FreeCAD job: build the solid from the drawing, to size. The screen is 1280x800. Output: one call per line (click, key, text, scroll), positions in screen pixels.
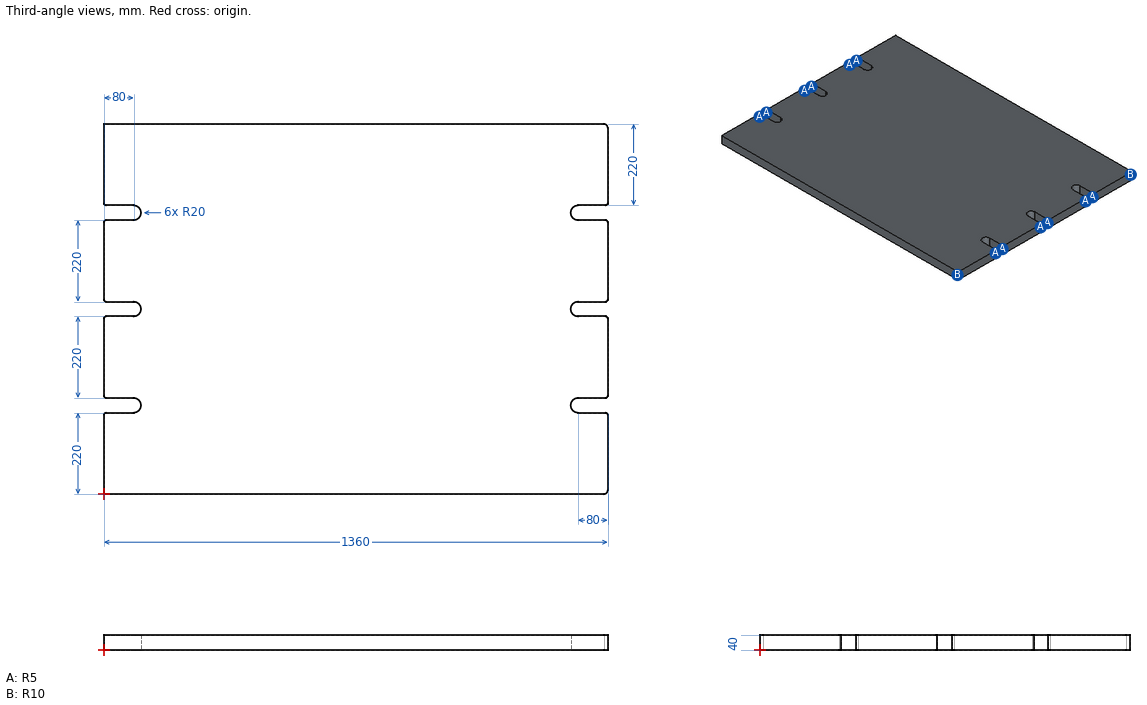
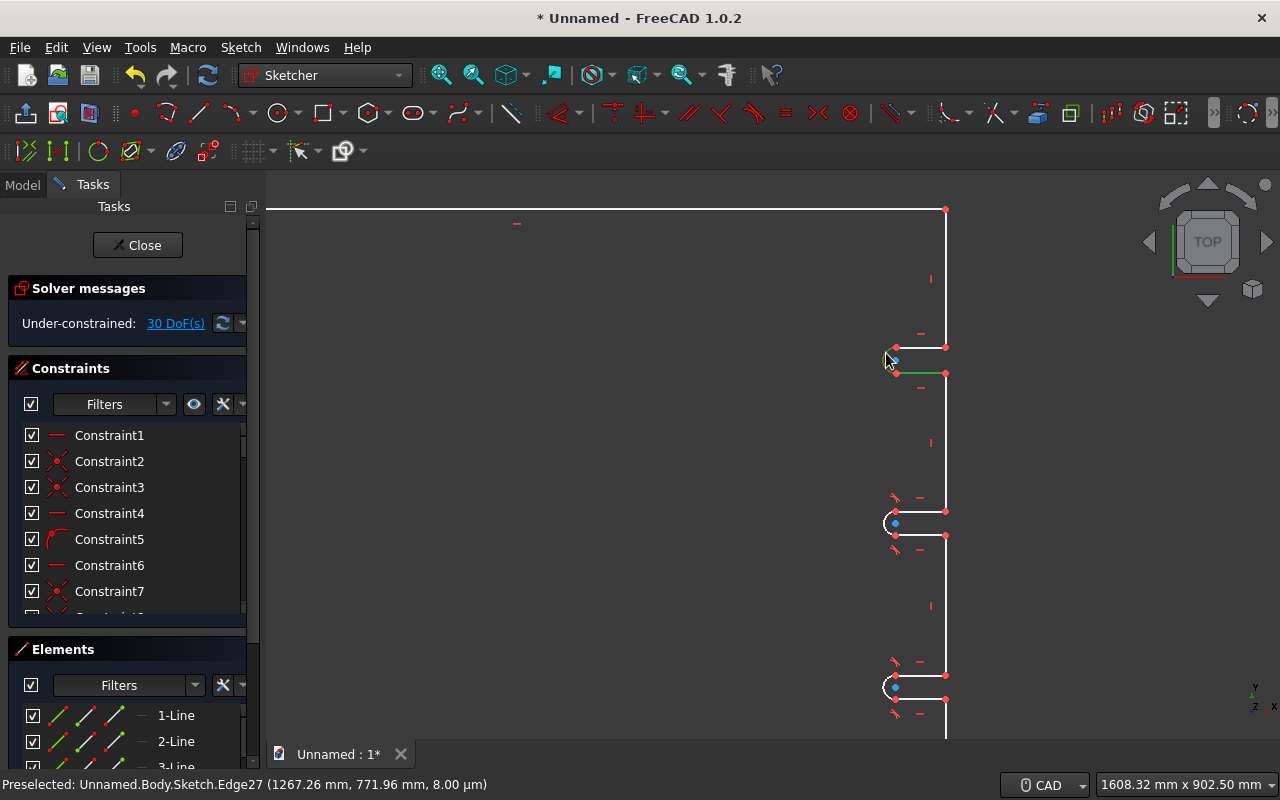
click(754, 114)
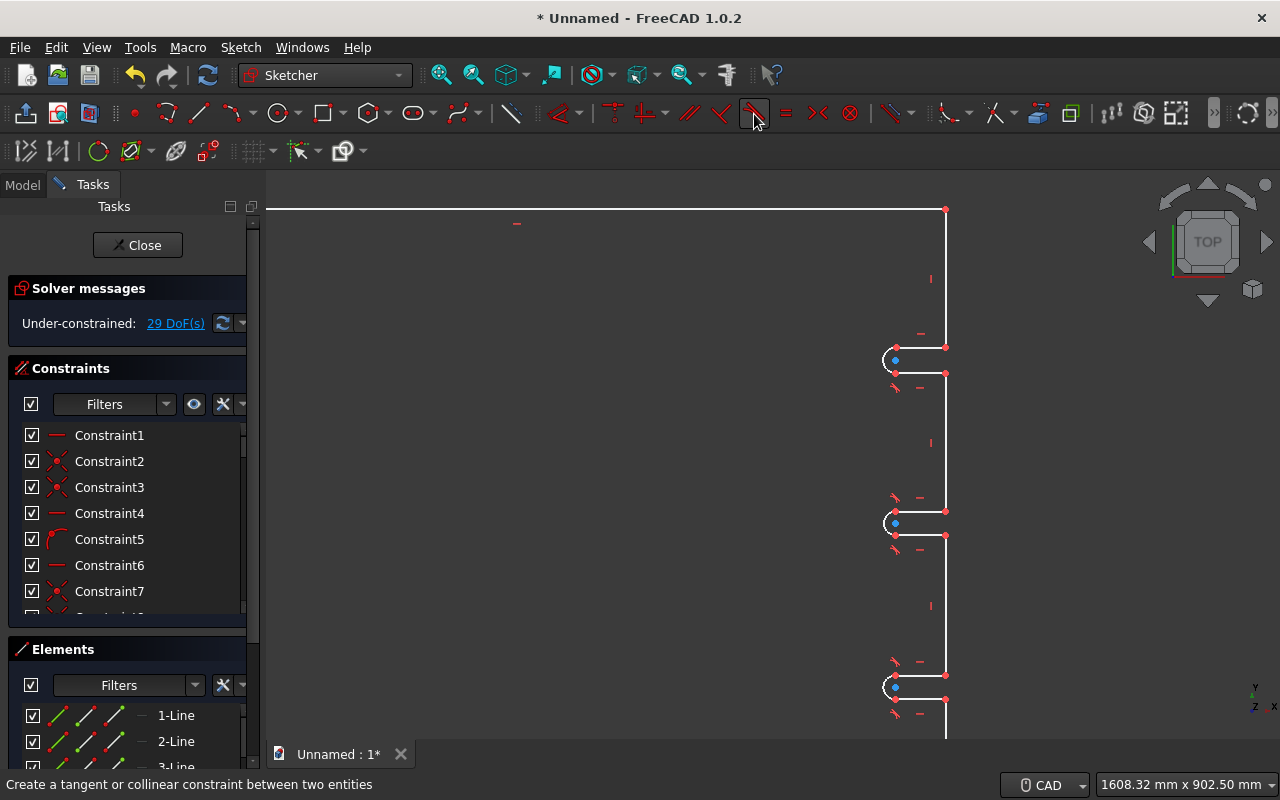
click(911, 348)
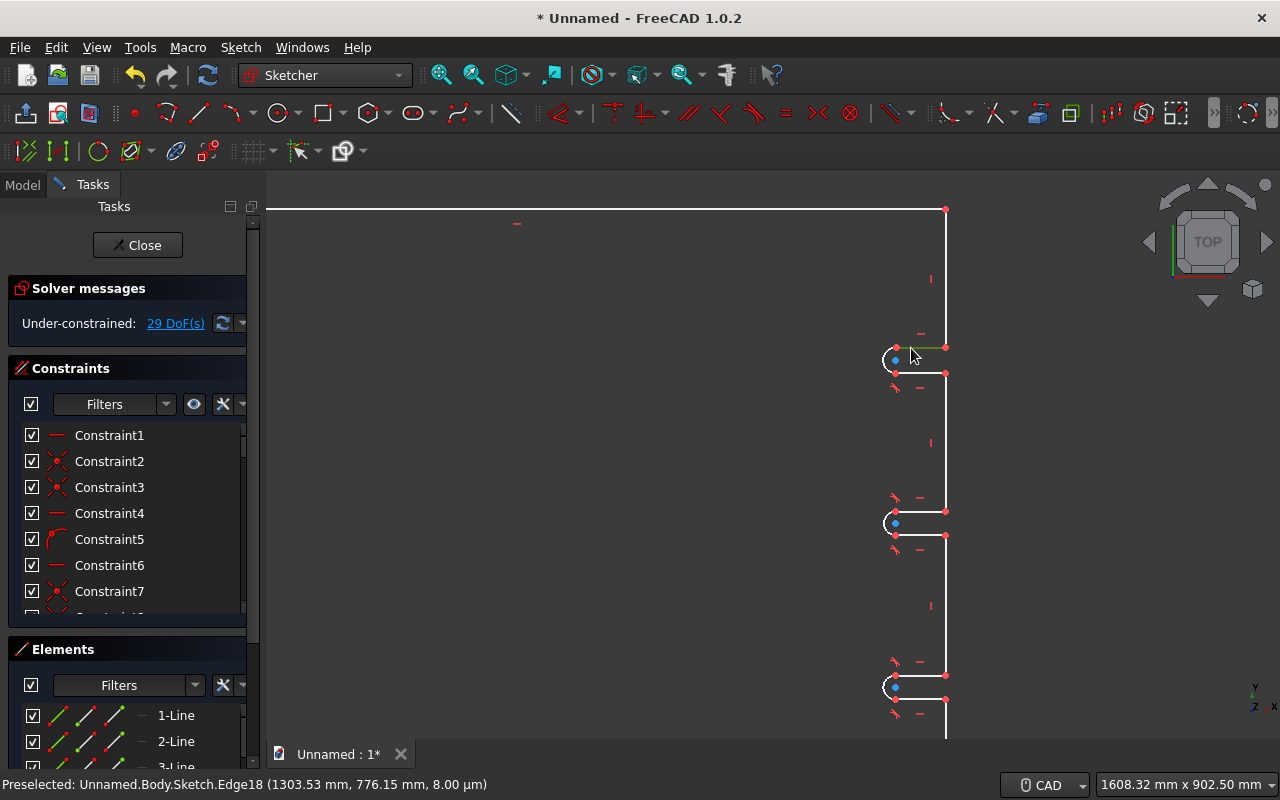
click(886, 352)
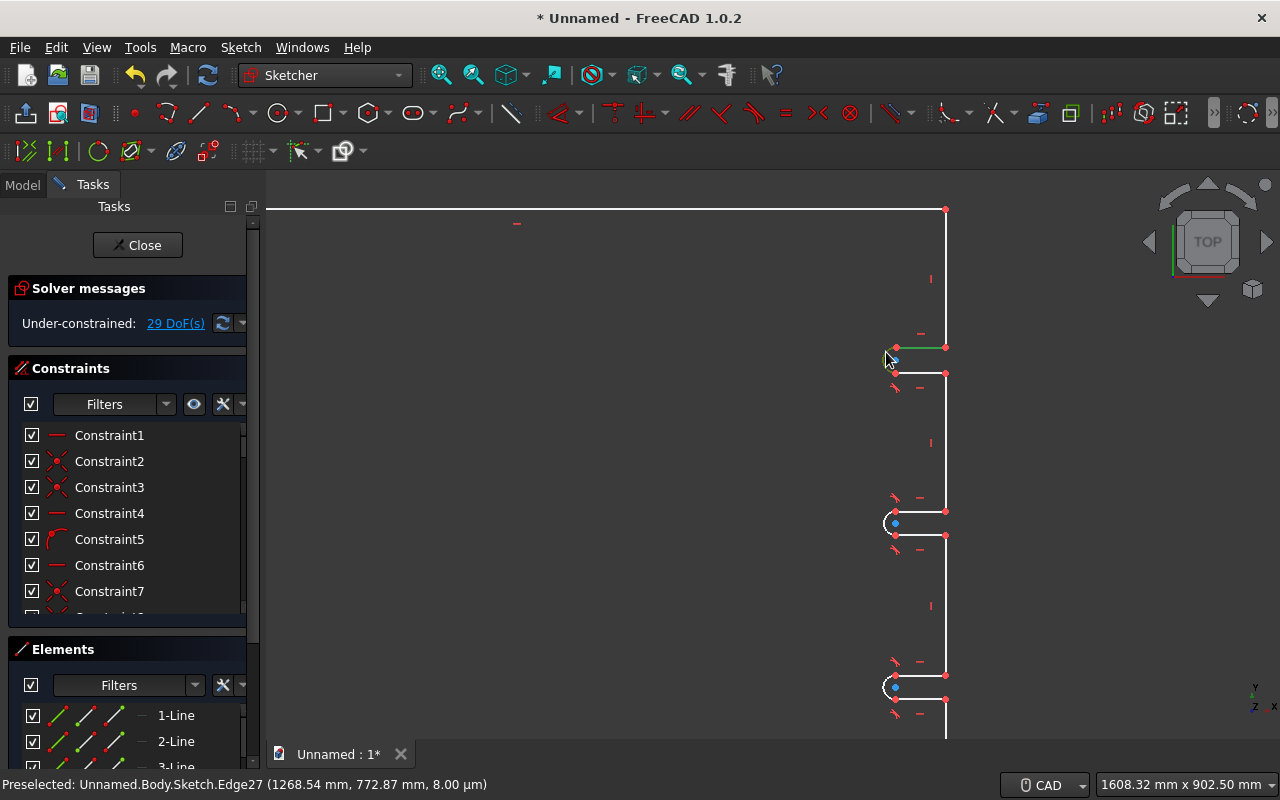
click(754, 114)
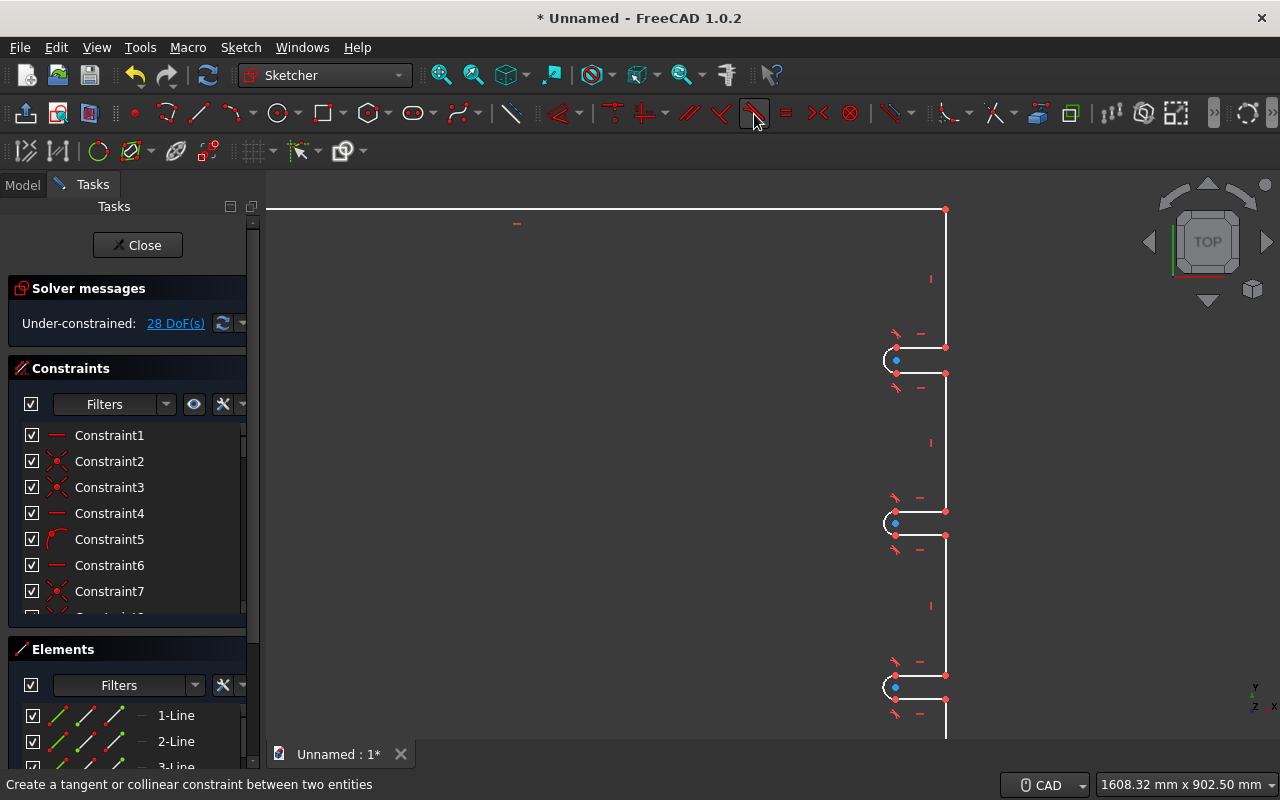
scroll(931, 373, down, 3)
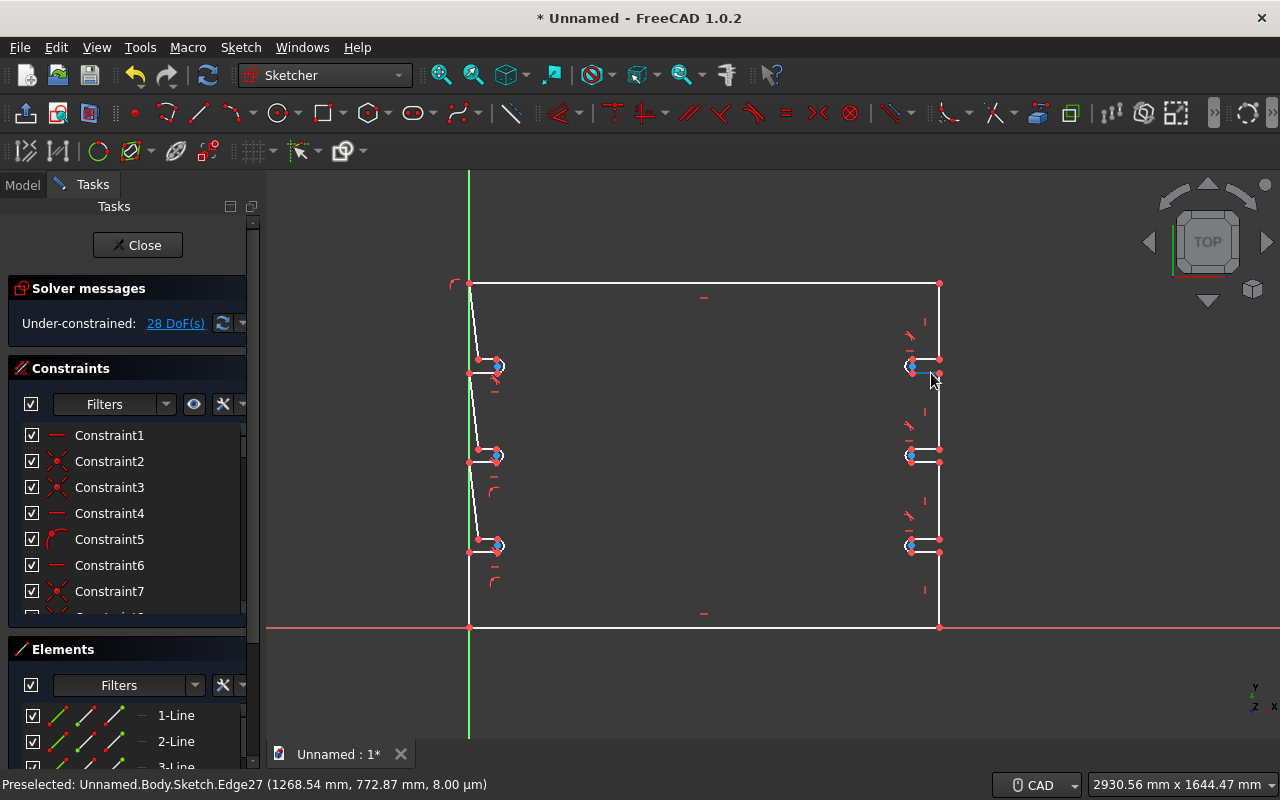
scroll(484, 359, up, 5)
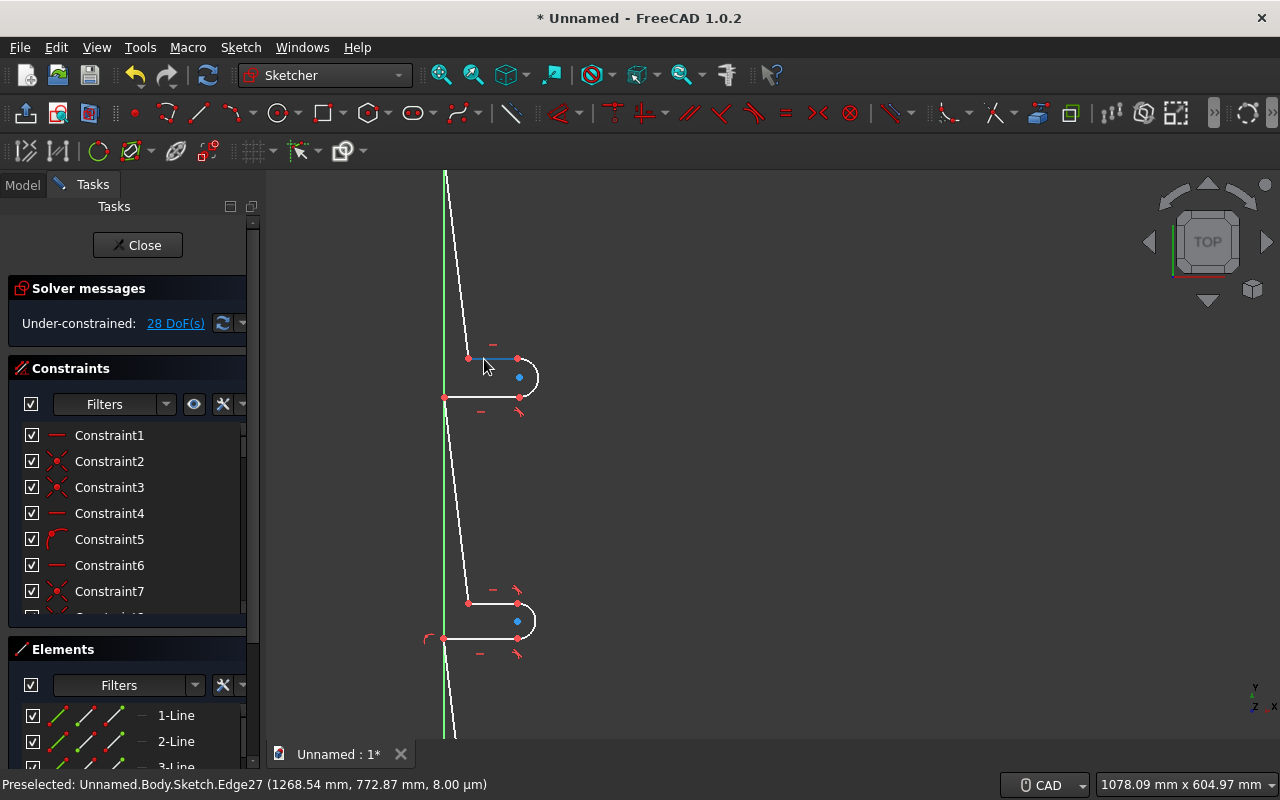
click(483, 359)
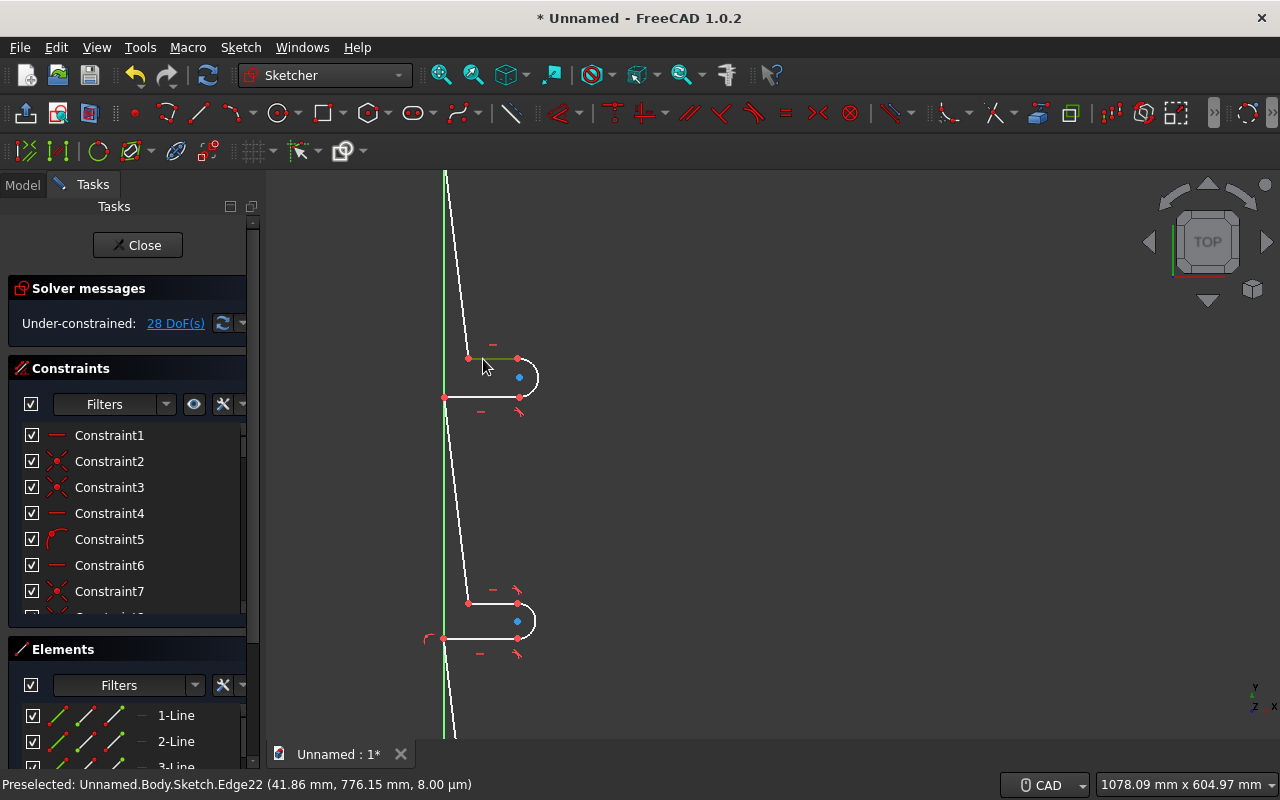
click(535, 389)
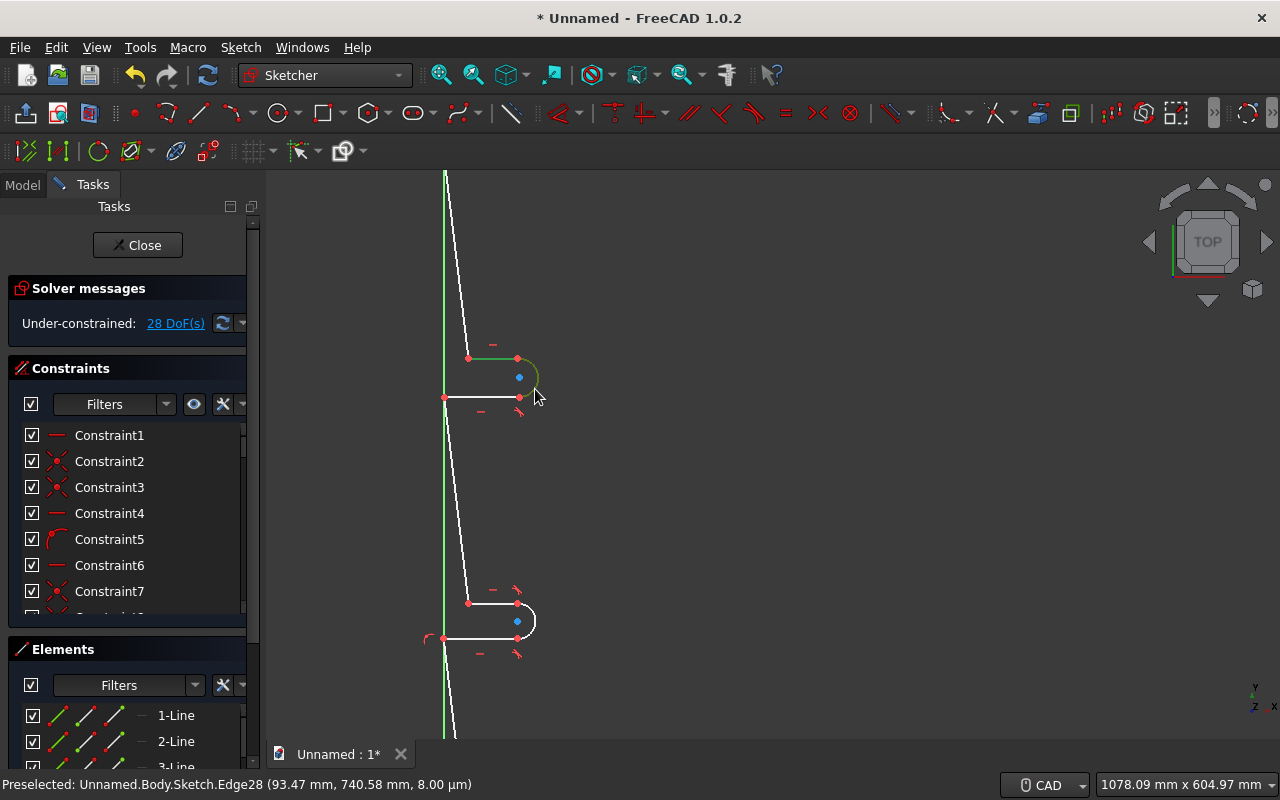
click(754, 114)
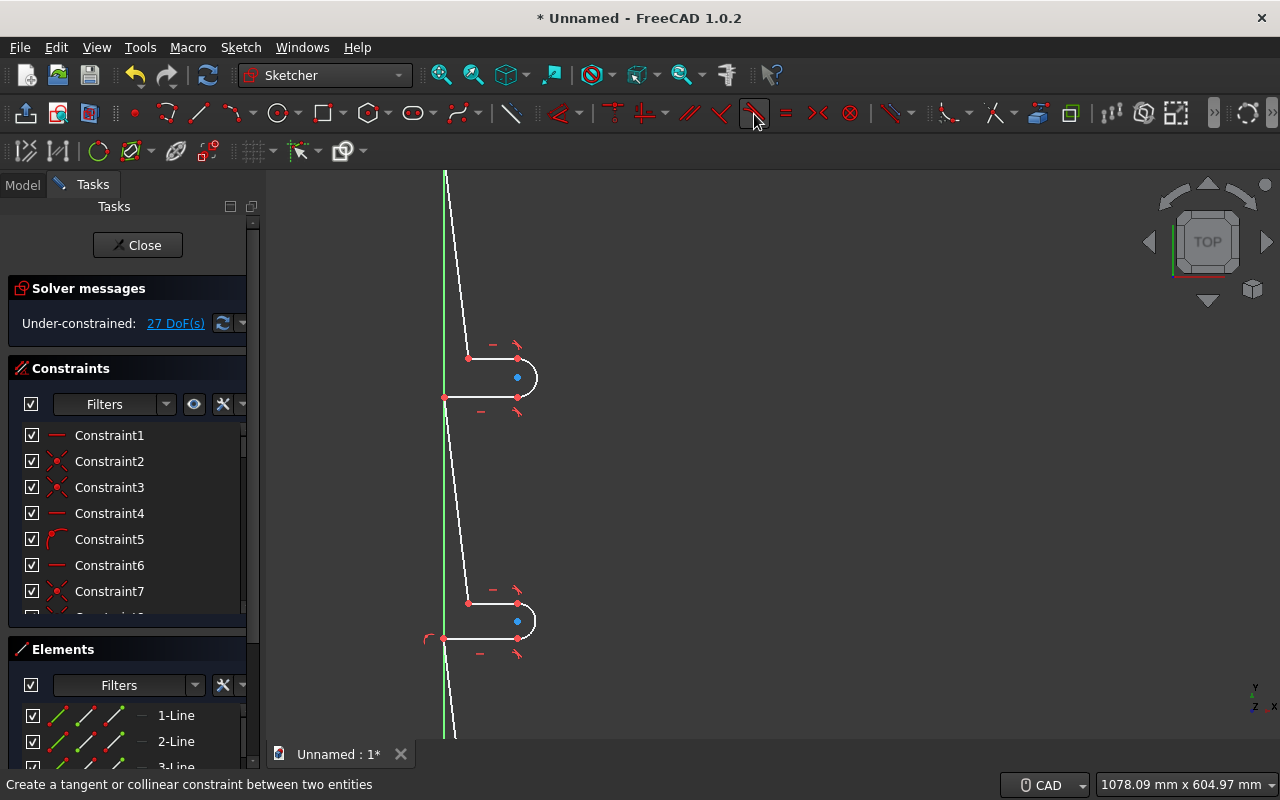
click(461, 542)